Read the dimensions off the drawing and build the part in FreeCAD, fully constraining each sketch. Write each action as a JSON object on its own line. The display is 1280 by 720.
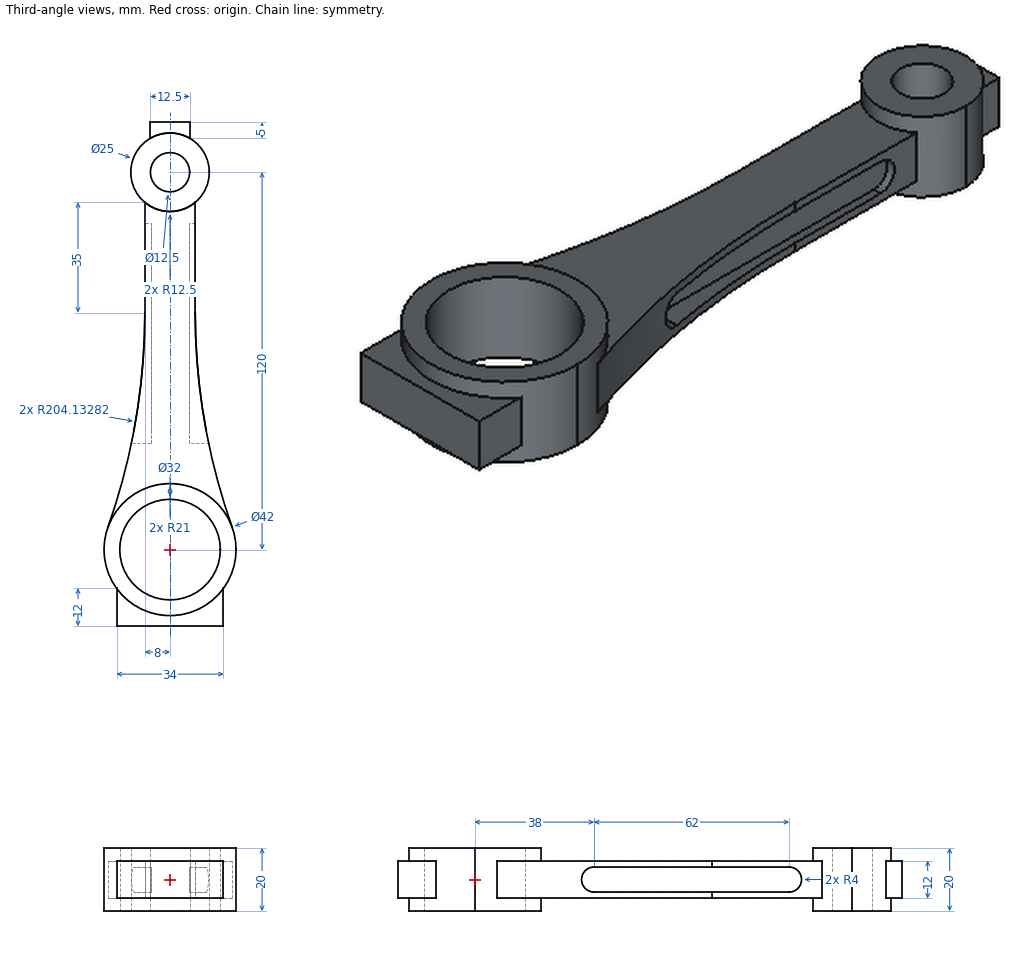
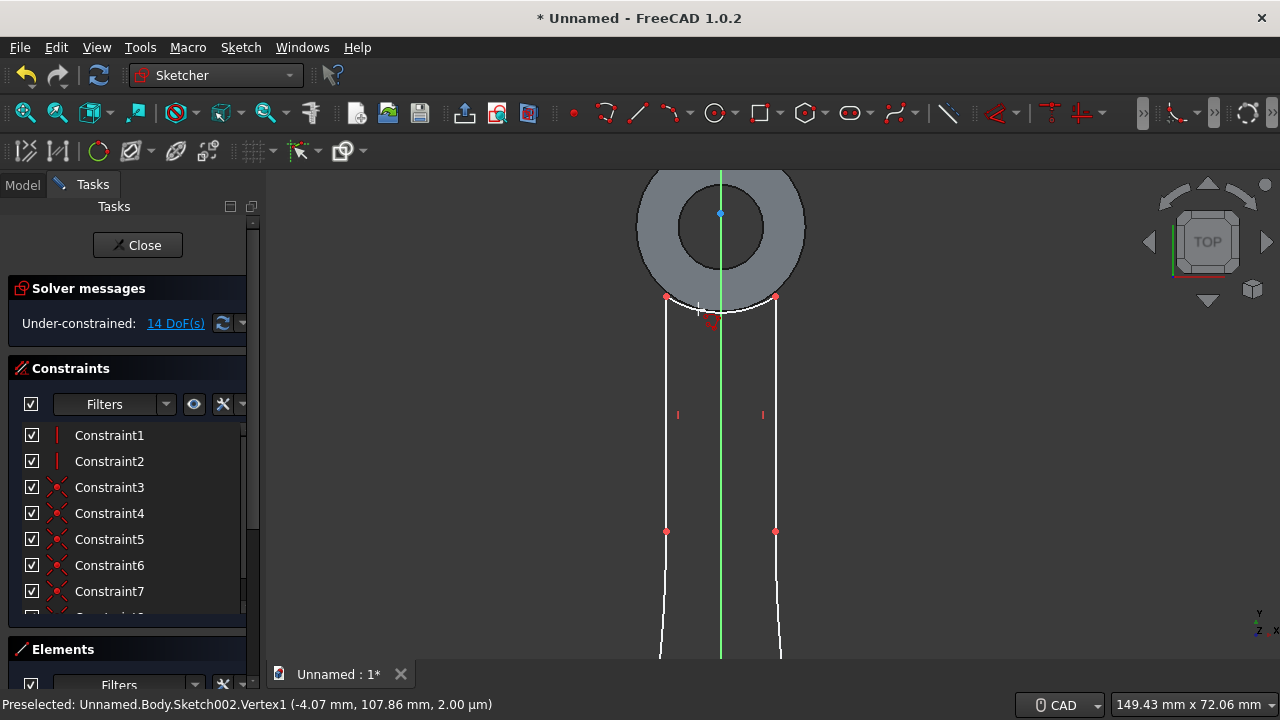
{"action": "scroll", "coordinate": [697, 307], "scroll_direction": "down", "scroll_amount": 6}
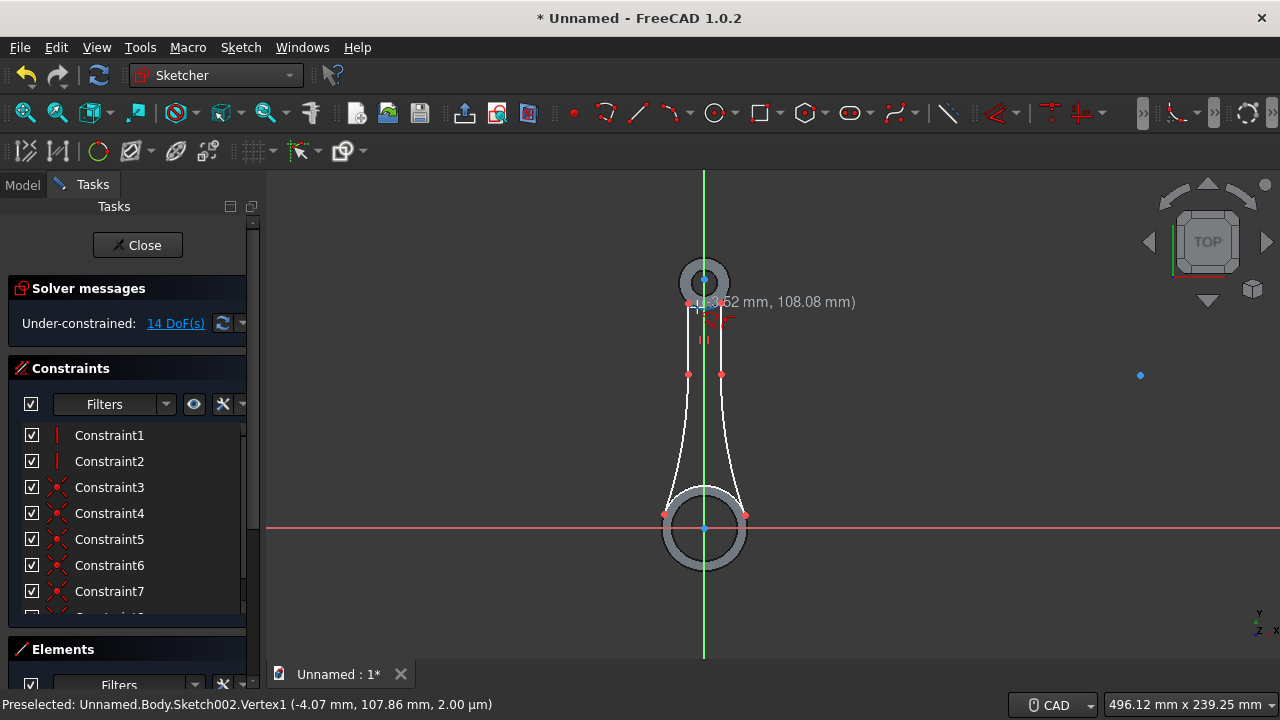
{"action": "scroll", "coordinate": [717, 261], "scroll_direction": "up", "scroll_amount": 2}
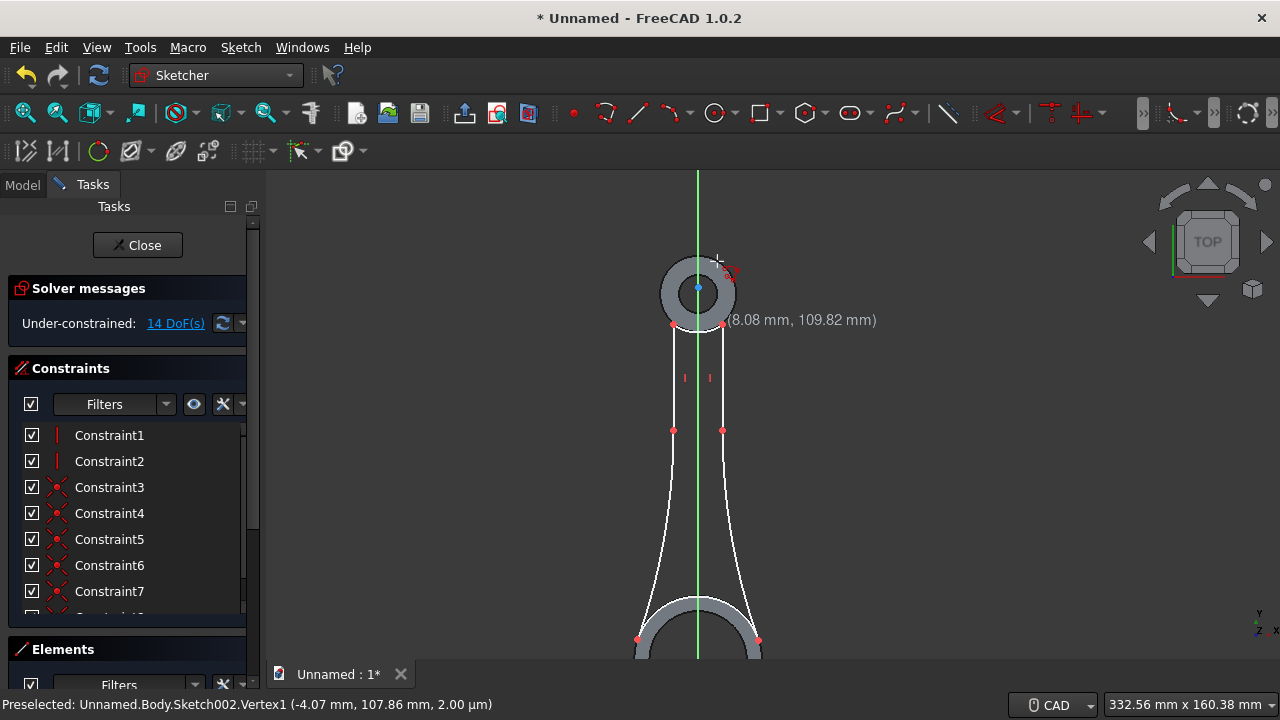
{"action": "left_click", "coordinate": [717, 261]}
{"action": "left_click", "coordinate": [717, 246]}
{"action": "left_click", "coordinate": [679, 246]}
{"action": "left_click", "coordinate": [679, 261]}
{"action": "right_click", "coordinate": [679, 261]}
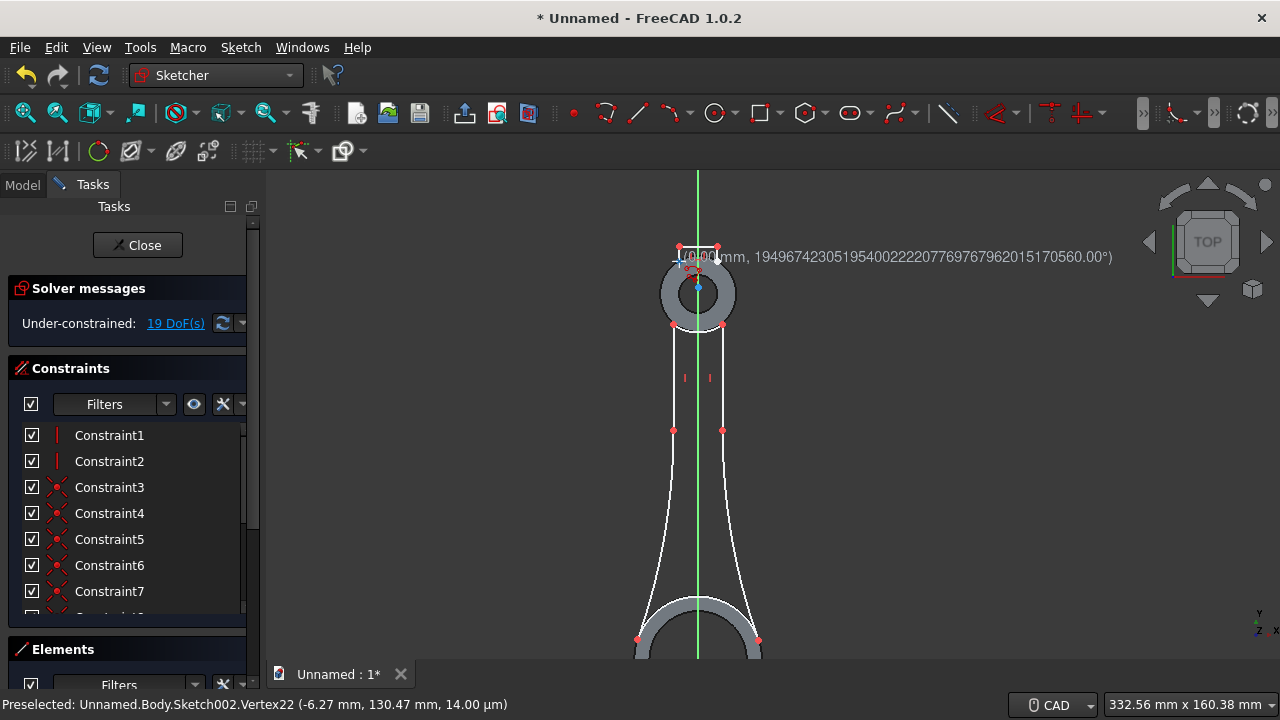
{"action": "key", "text": "g 3 a"}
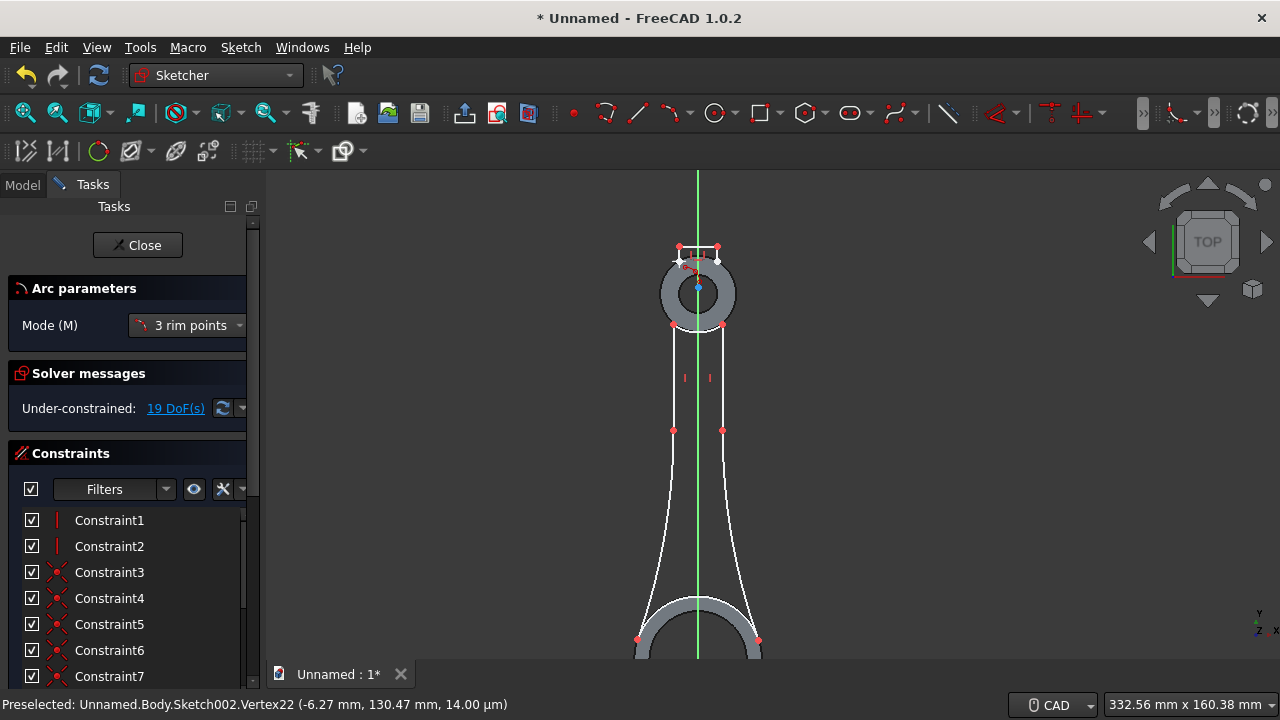
{"action": "scroll", "coordinate": [679, 261], "scroll_direction": "up", "scroll_amount": 4}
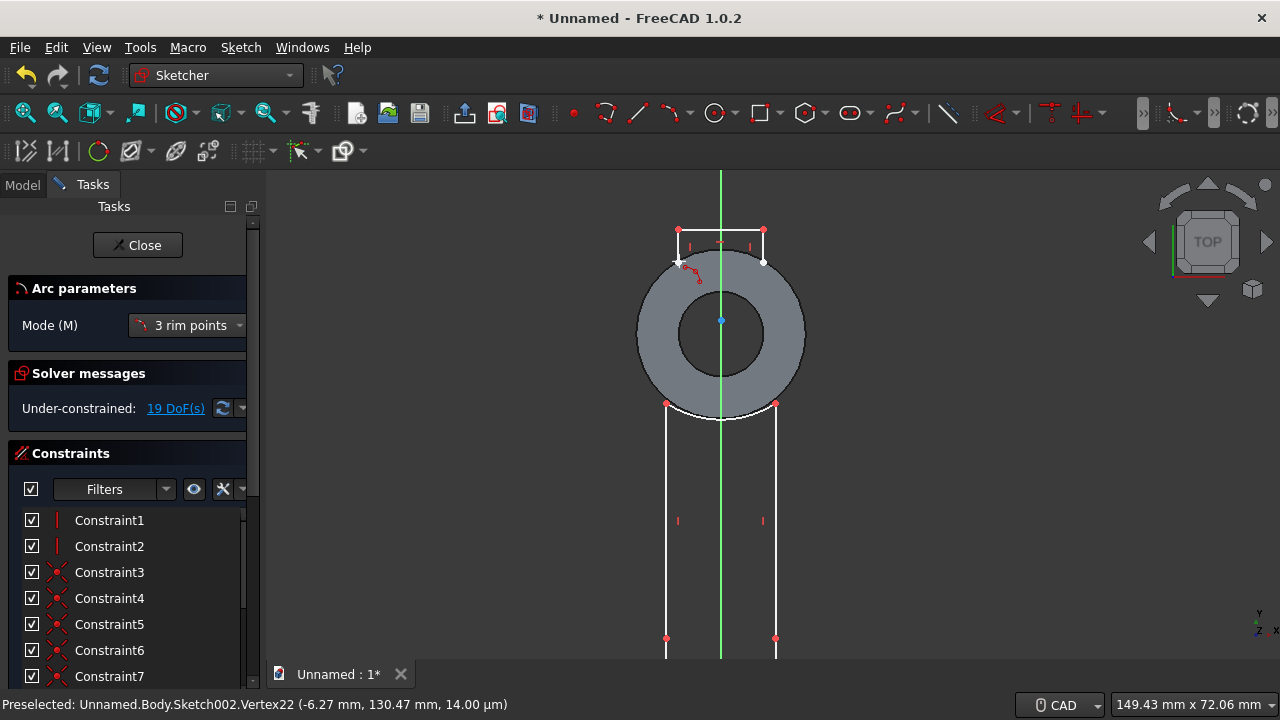
{"action": "left_click", "coordinate": [679, 263]}
{"action": "left_click", "coordinate": [763, 263]}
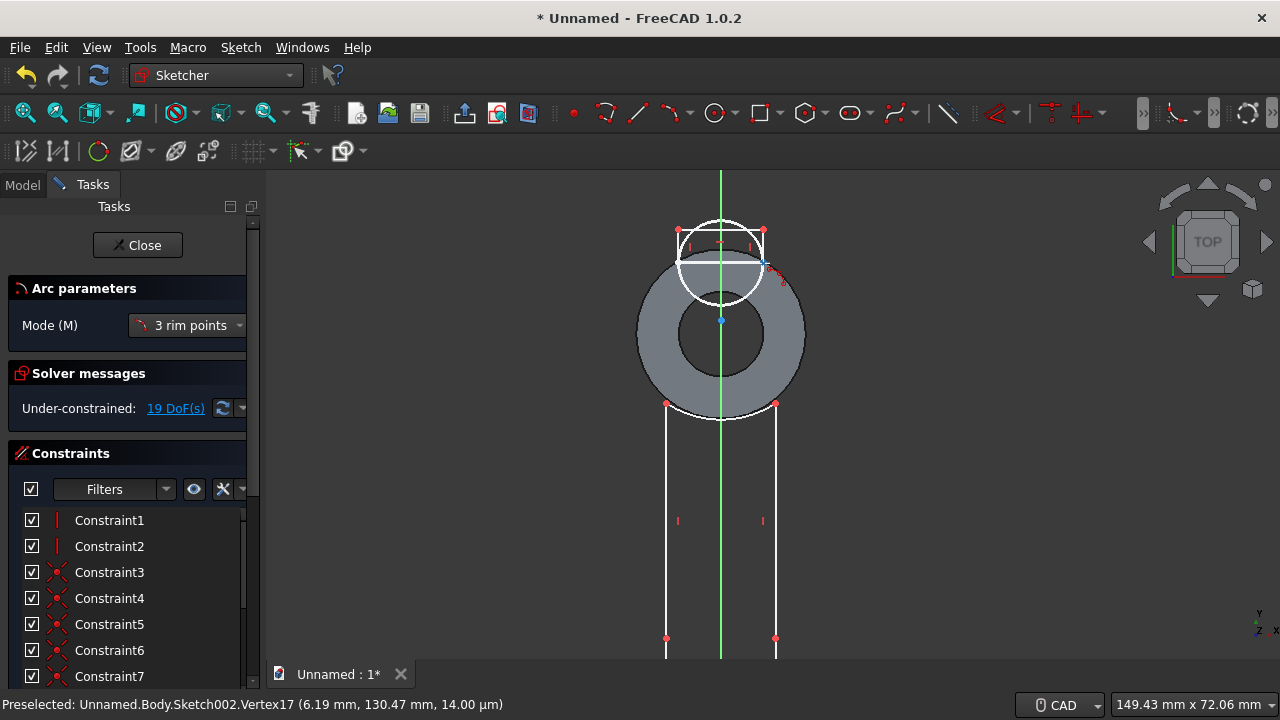
{"action": "scroll", "coordinate": [739, 251], "scroll_direction": "up", "scroll_amount": 3}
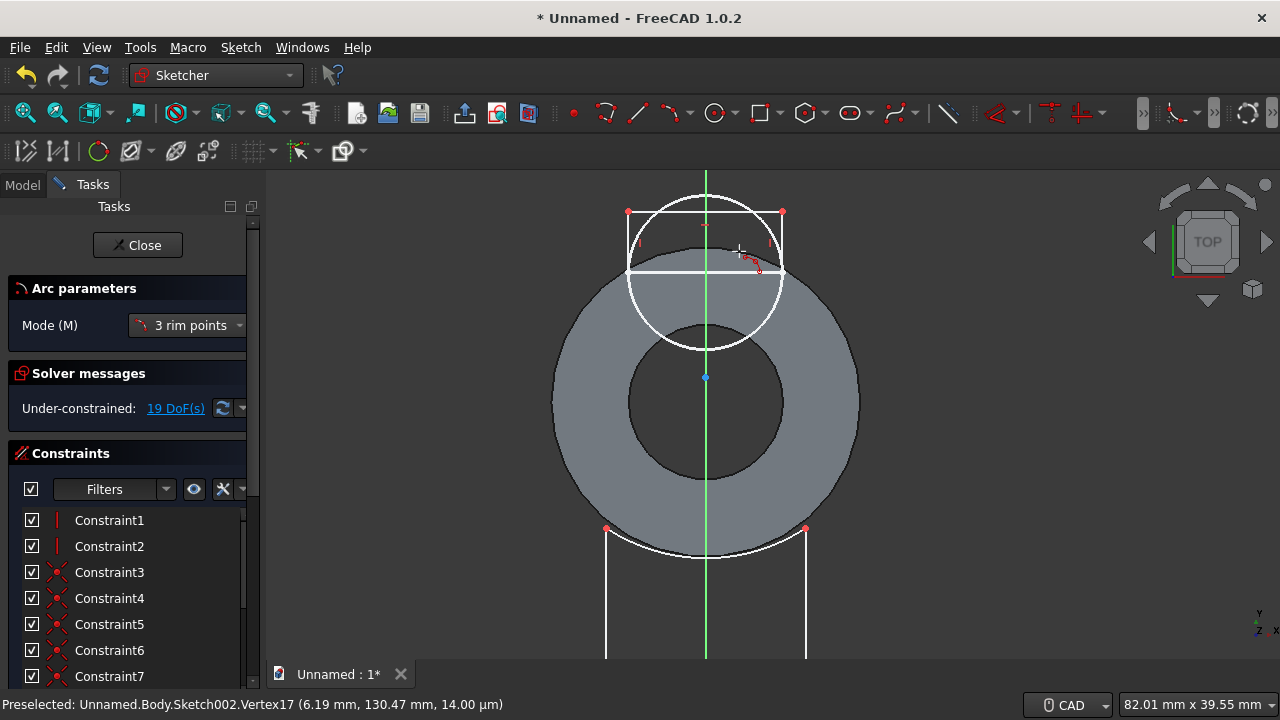
{"action": "left_click", "coordinate": [738, 251]}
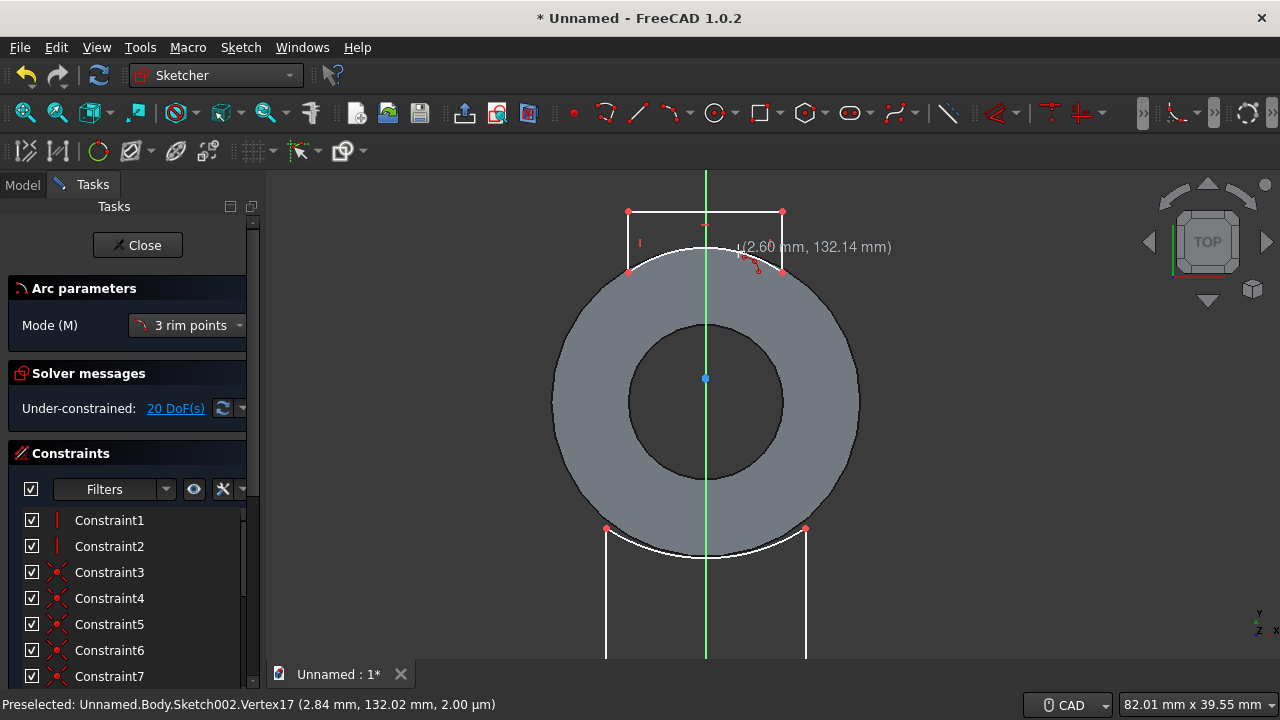
{"action": "key", "text": "g m"}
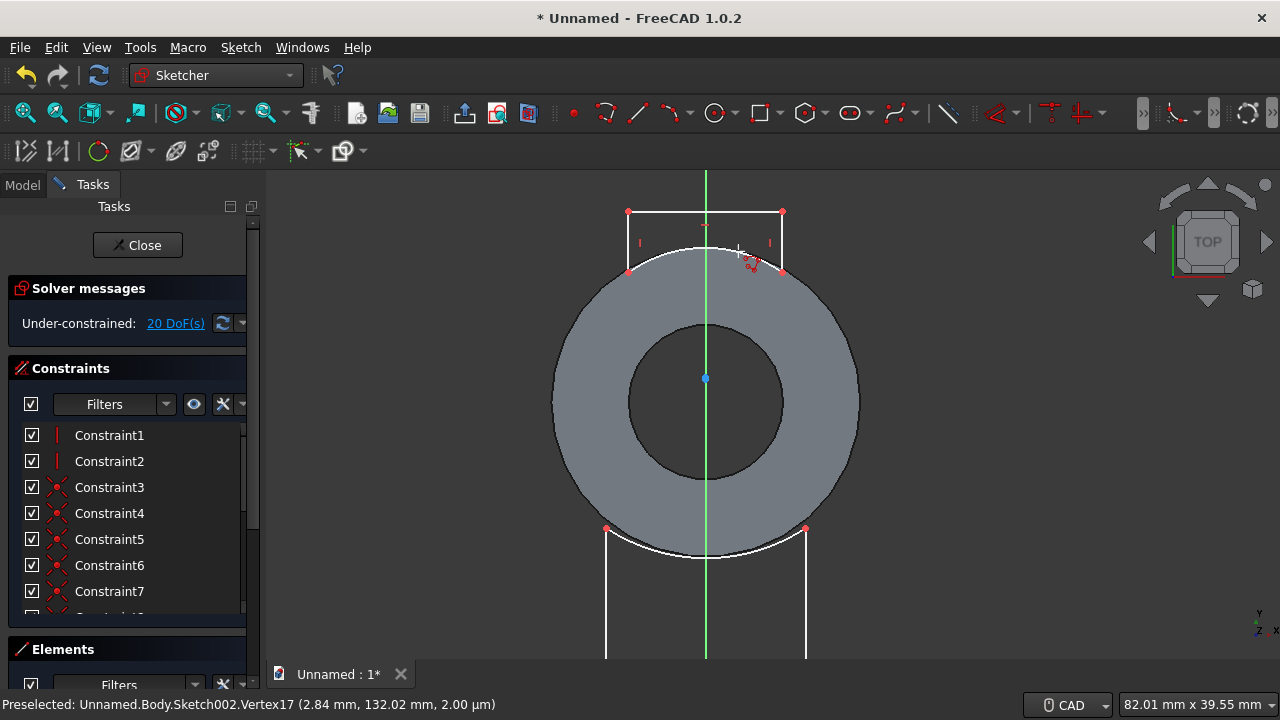
{"action": "scroll", "coordinate": [704, 260], "scroll_direction": "down", "scroll_amount": 9}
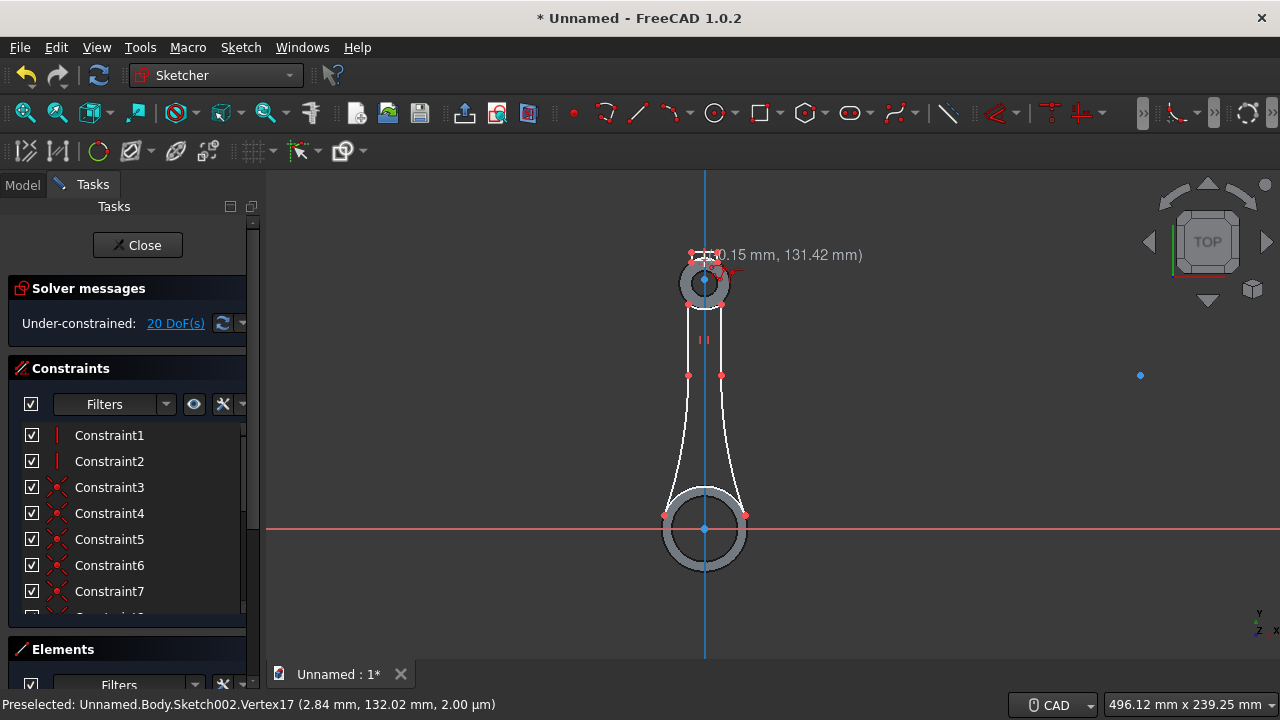
{"action": "left_click", "coordinate": [670, 554]}
{"action": "left_click", "coordinate": [670, 579]}
{"action": "left_click", "coordinate": [739, 579]}
{"action": "left_click", "coordinate": [739, 554]}
{"action": "right_click", "coordinate": [739, 554]}